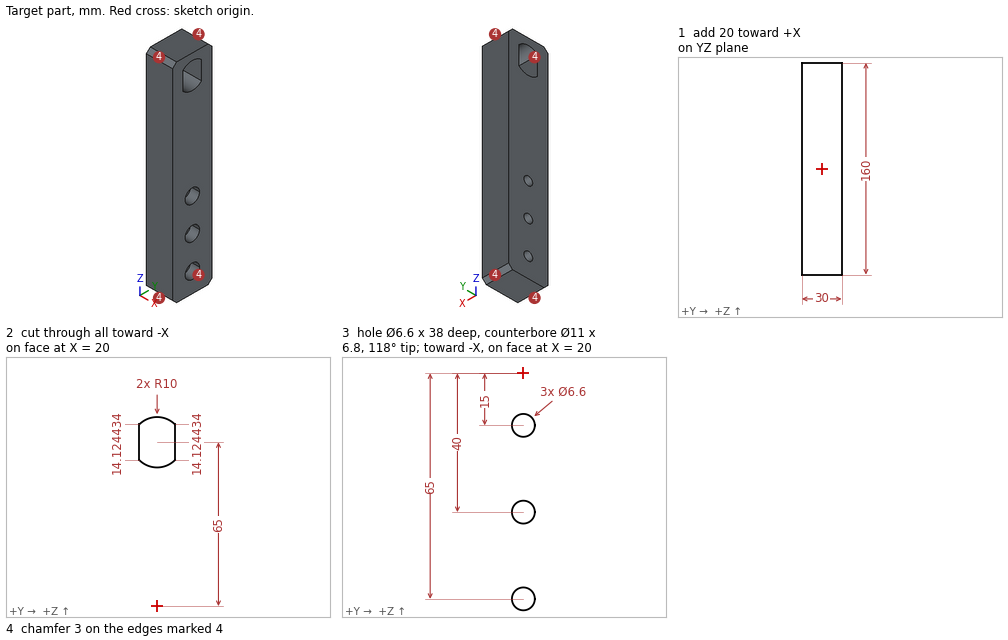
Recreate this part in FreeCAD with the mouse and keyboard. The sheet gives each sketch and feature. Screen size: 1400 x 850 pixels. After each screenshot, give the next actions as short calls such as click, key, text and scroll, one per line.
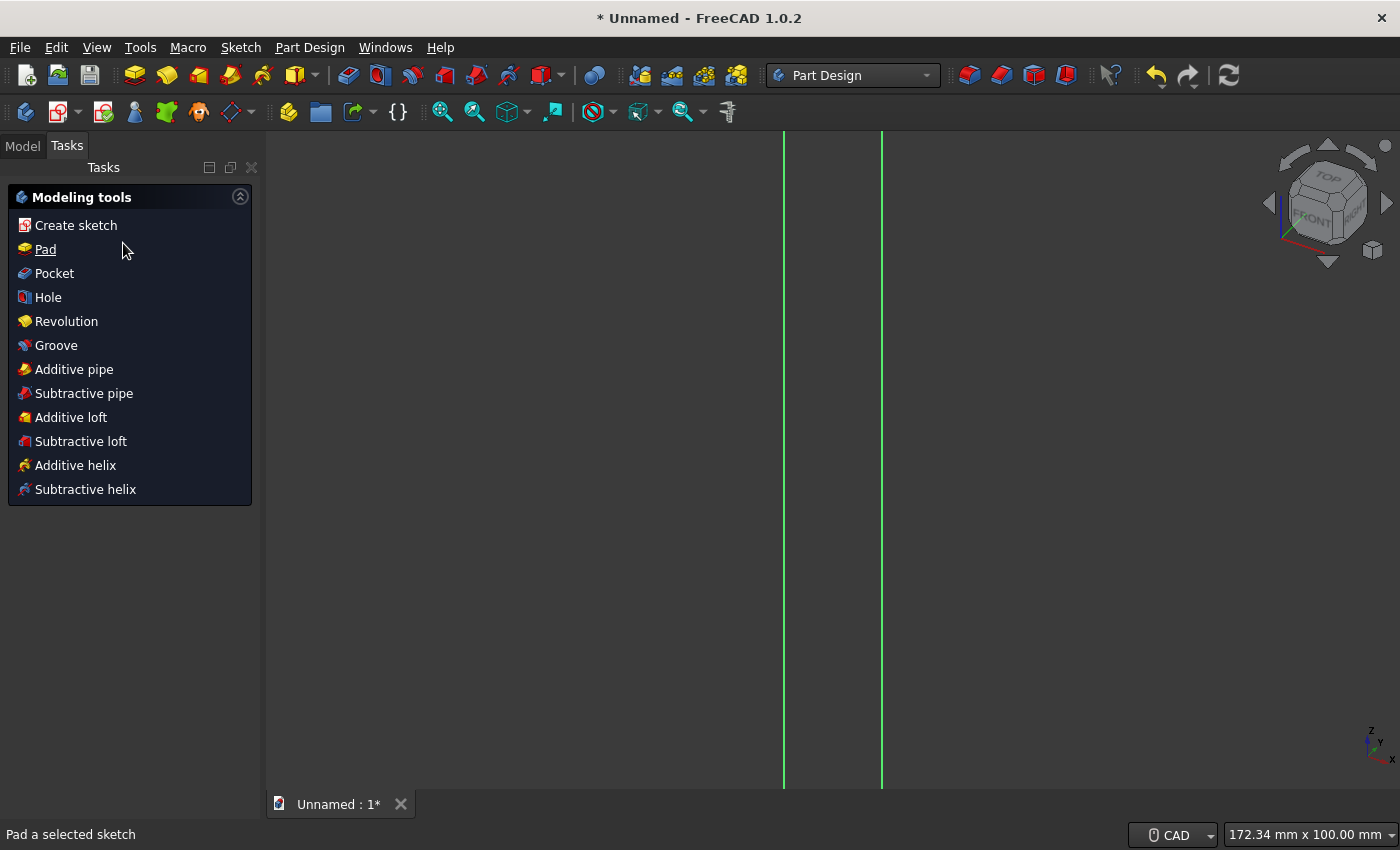
click(136, 76)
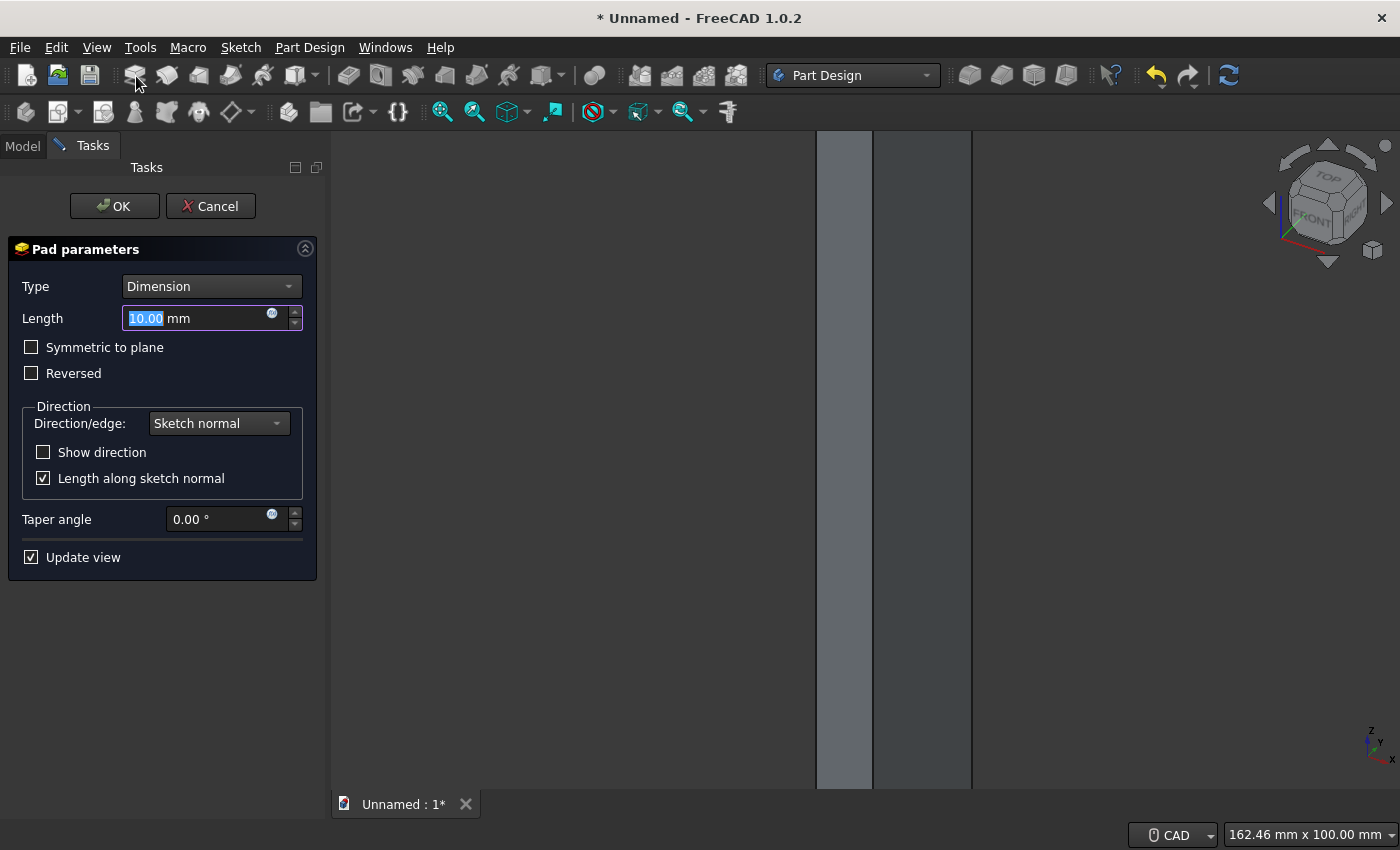
text(20)
key(Tab)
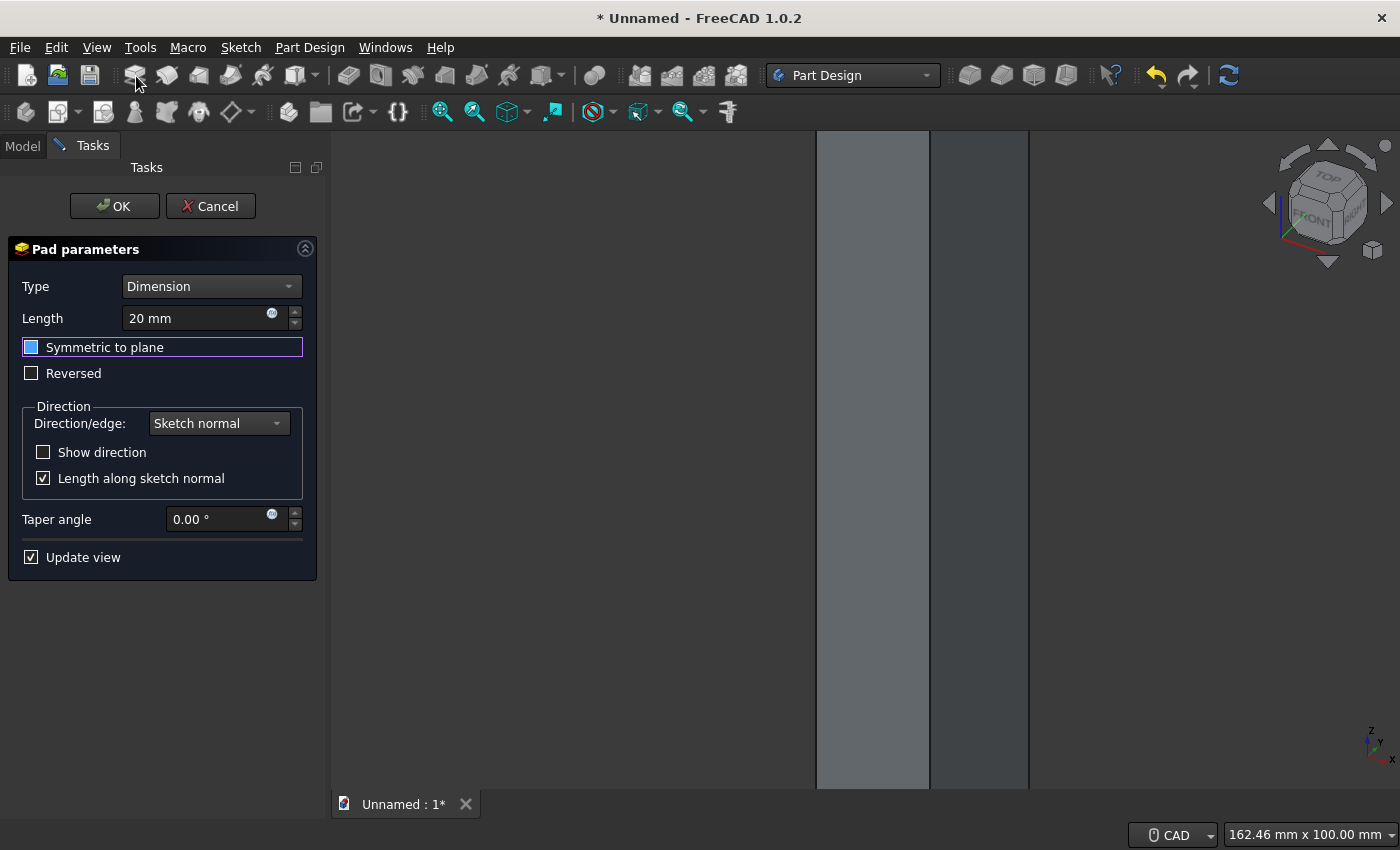
click(115, 206)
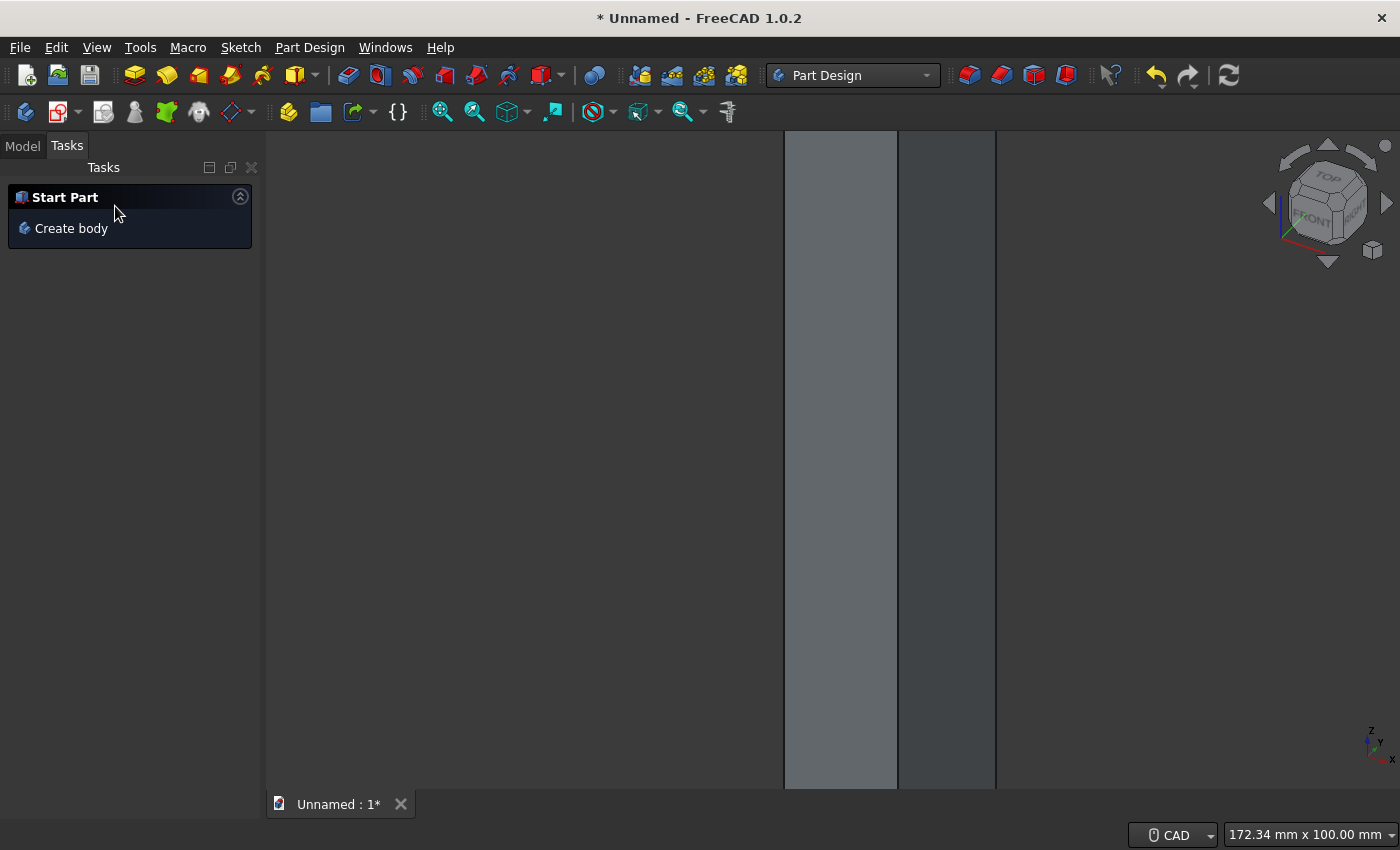
click(444, 112)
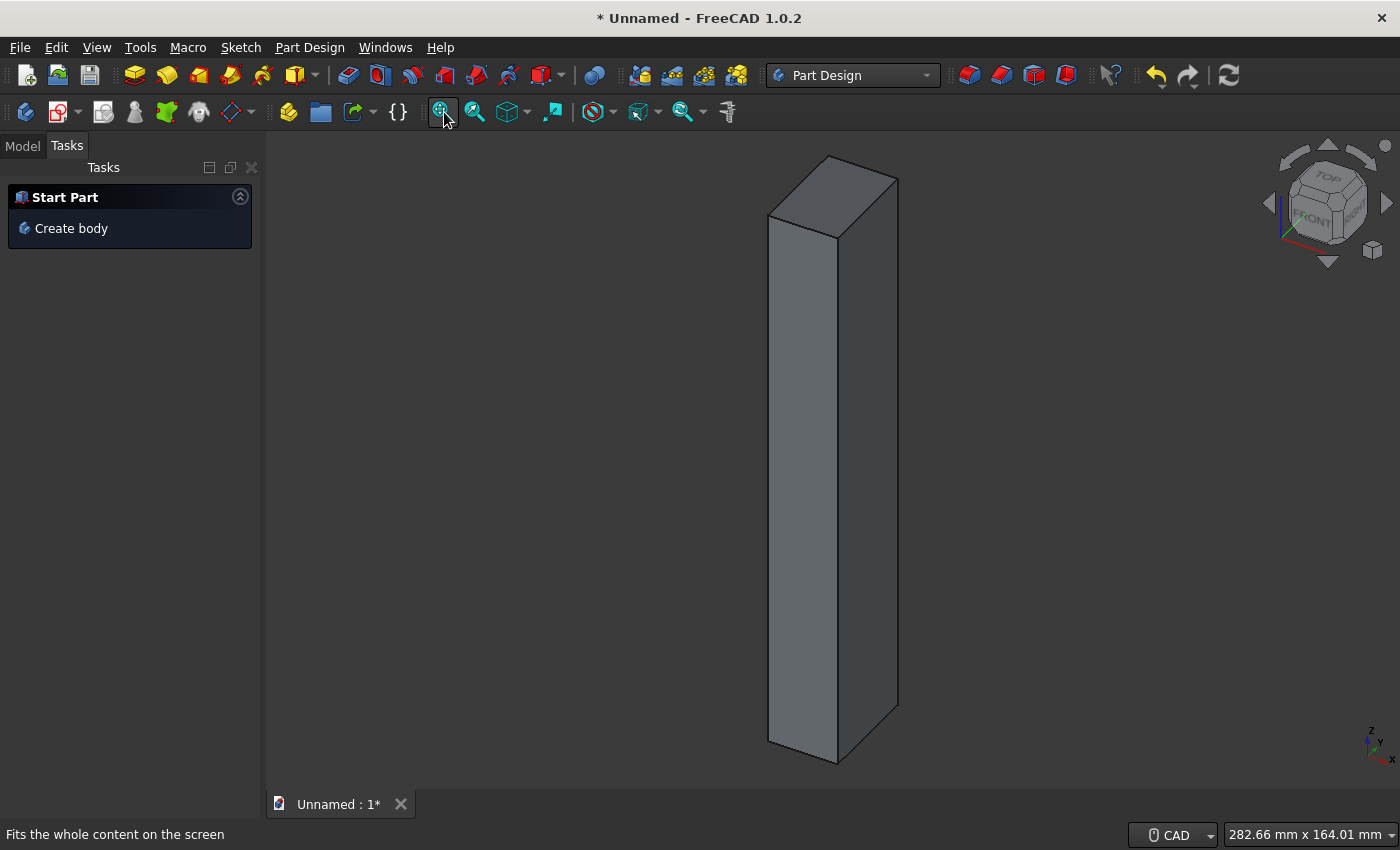
click(868, 621)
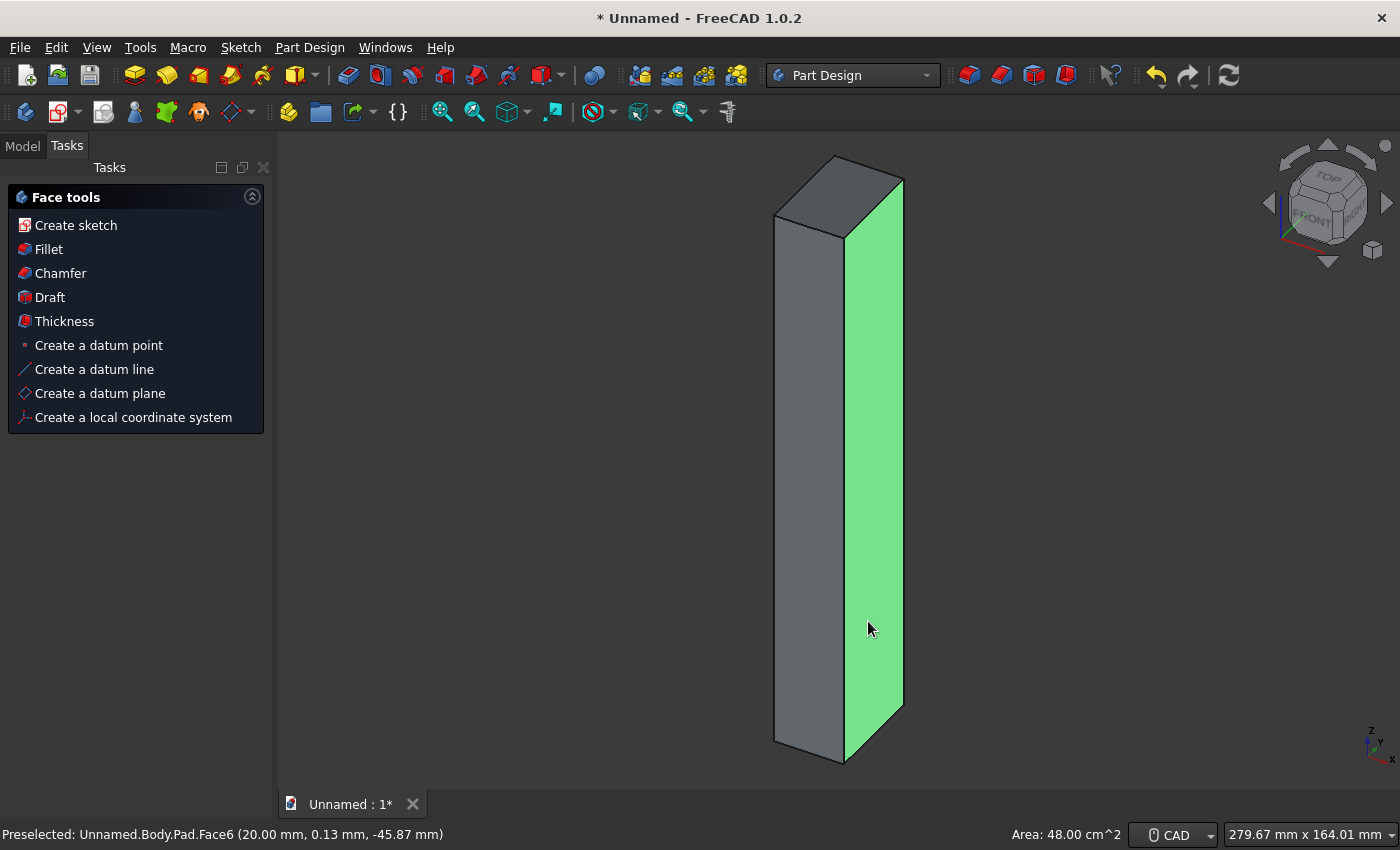
click(58, 112)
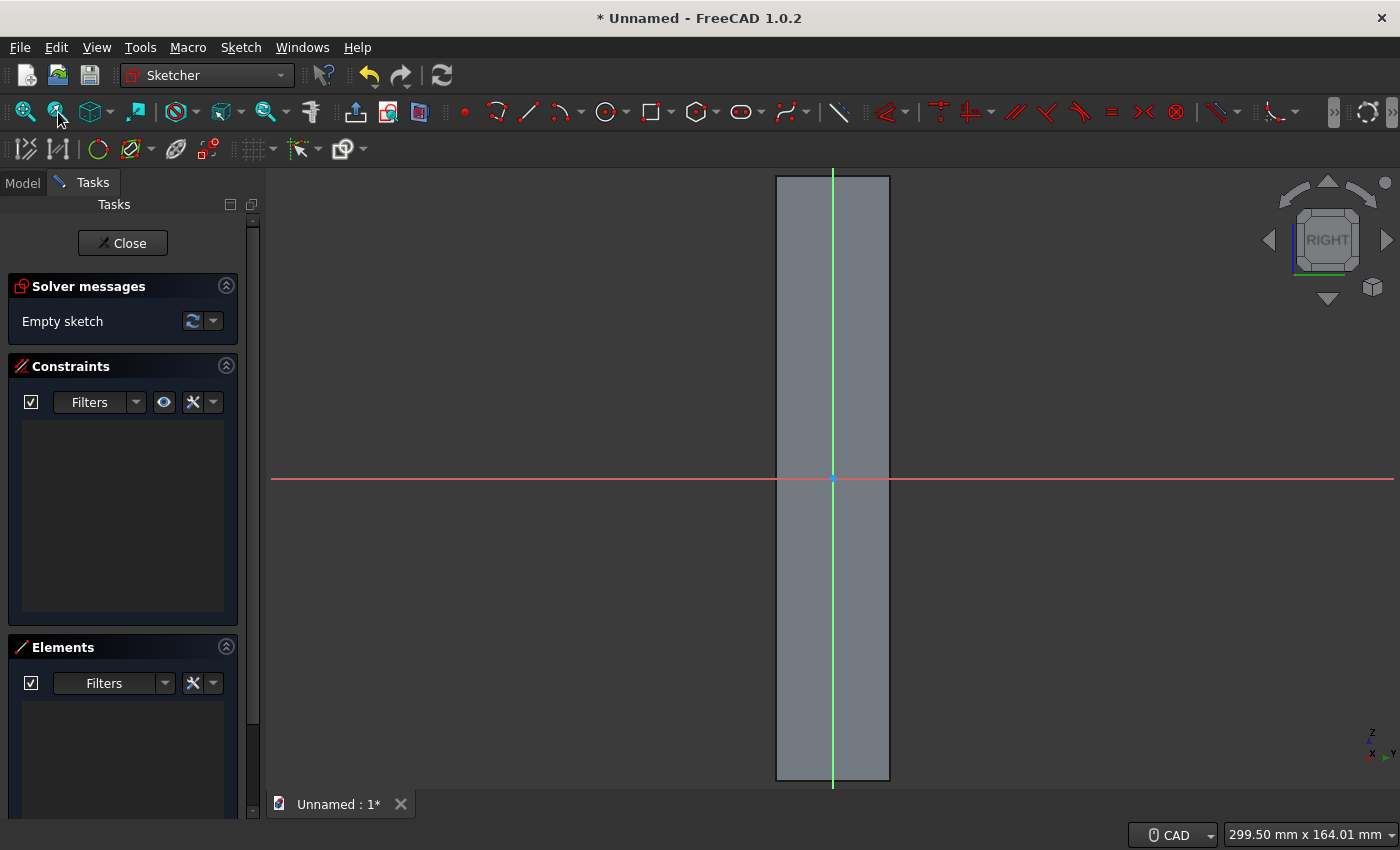
scroll(764, 478, down, 5)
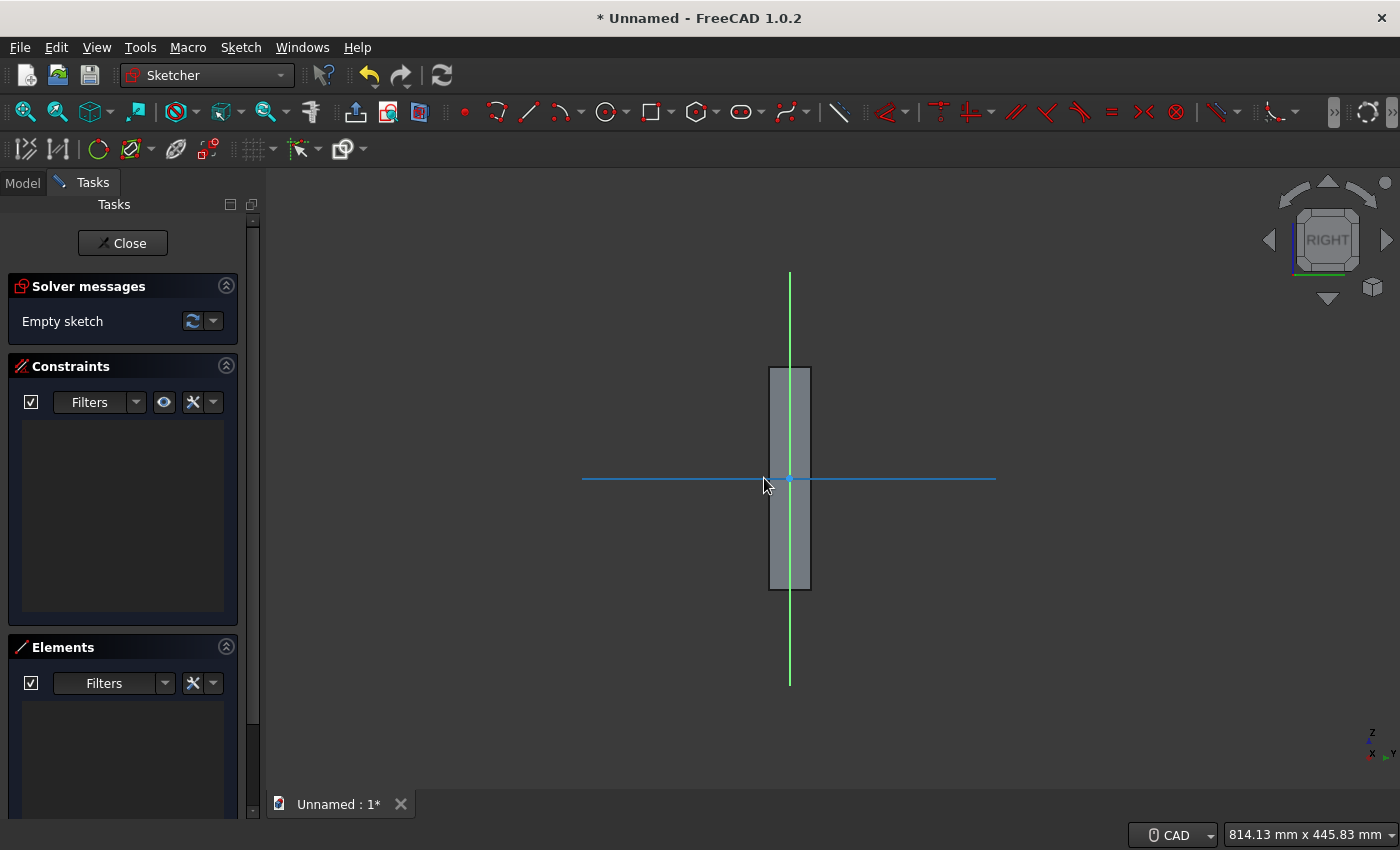
scroll(792, 381, up, 13)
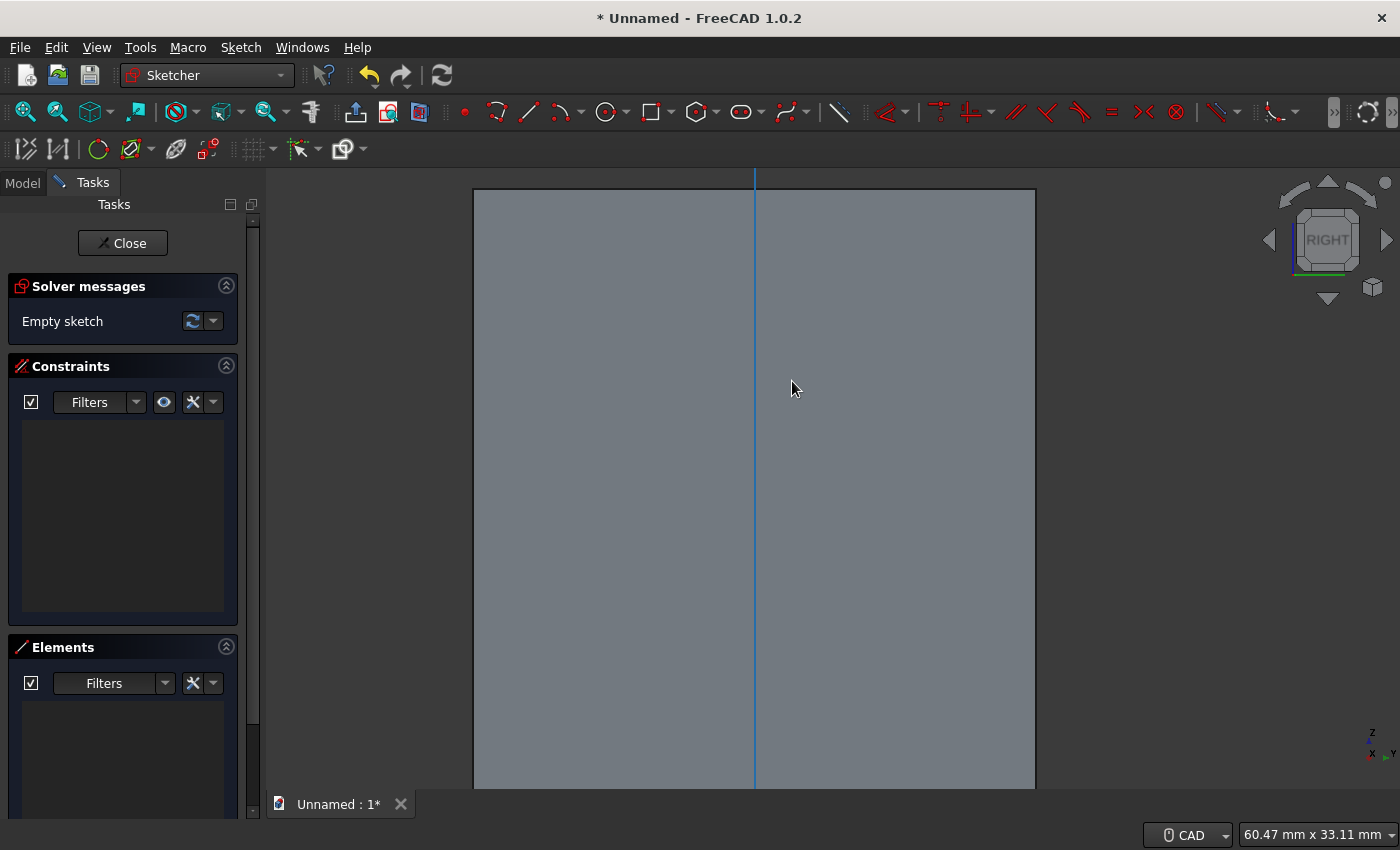
key(g)
key(l)